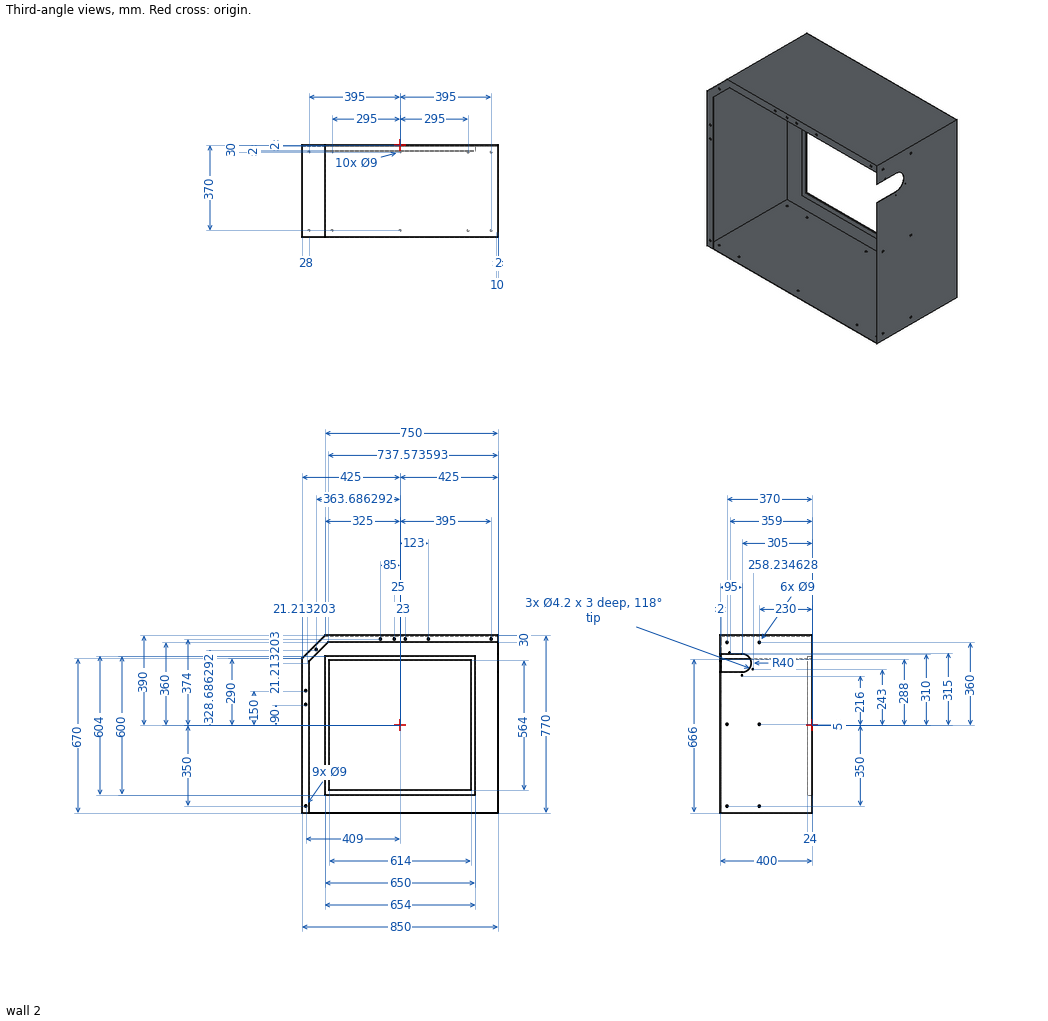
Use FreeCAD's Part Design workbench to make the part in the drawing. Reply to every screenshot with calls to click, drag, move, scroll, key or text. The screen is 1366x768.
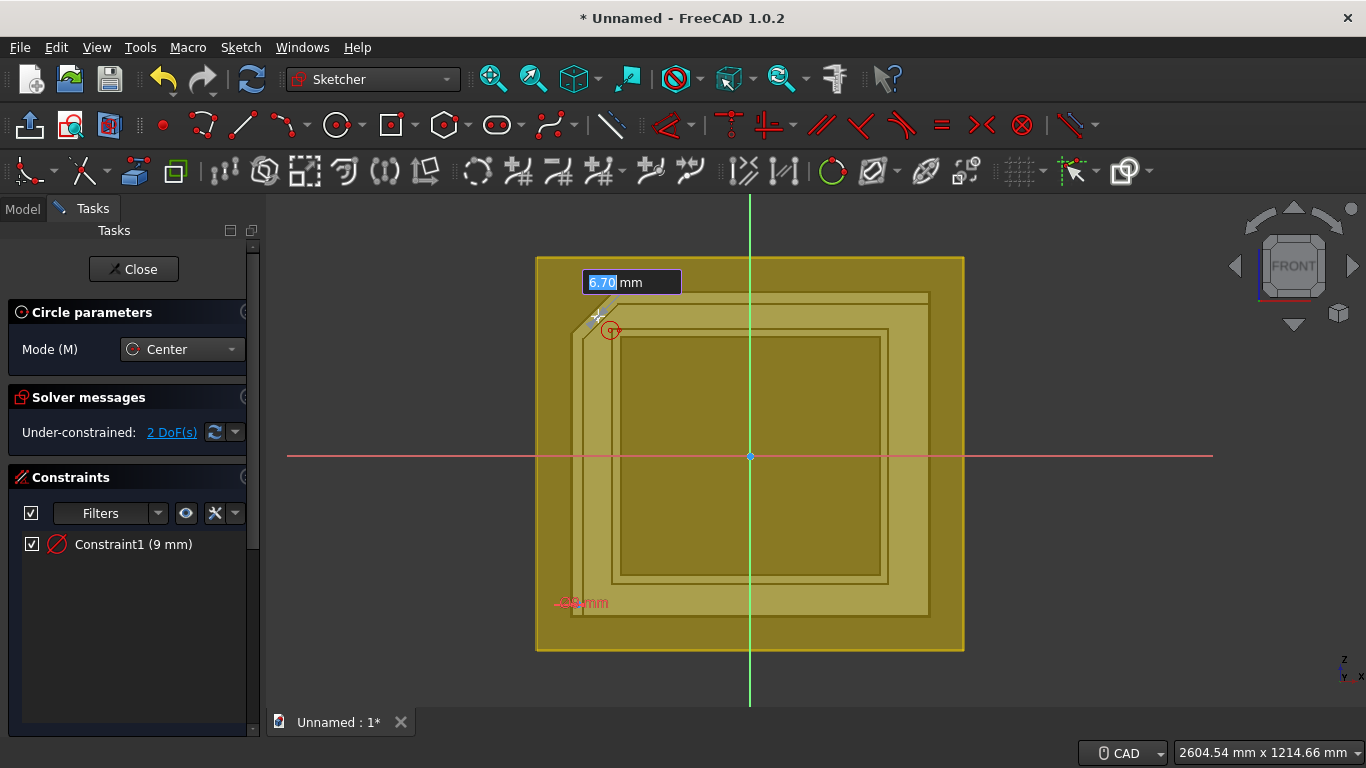
text(9)
key(Return)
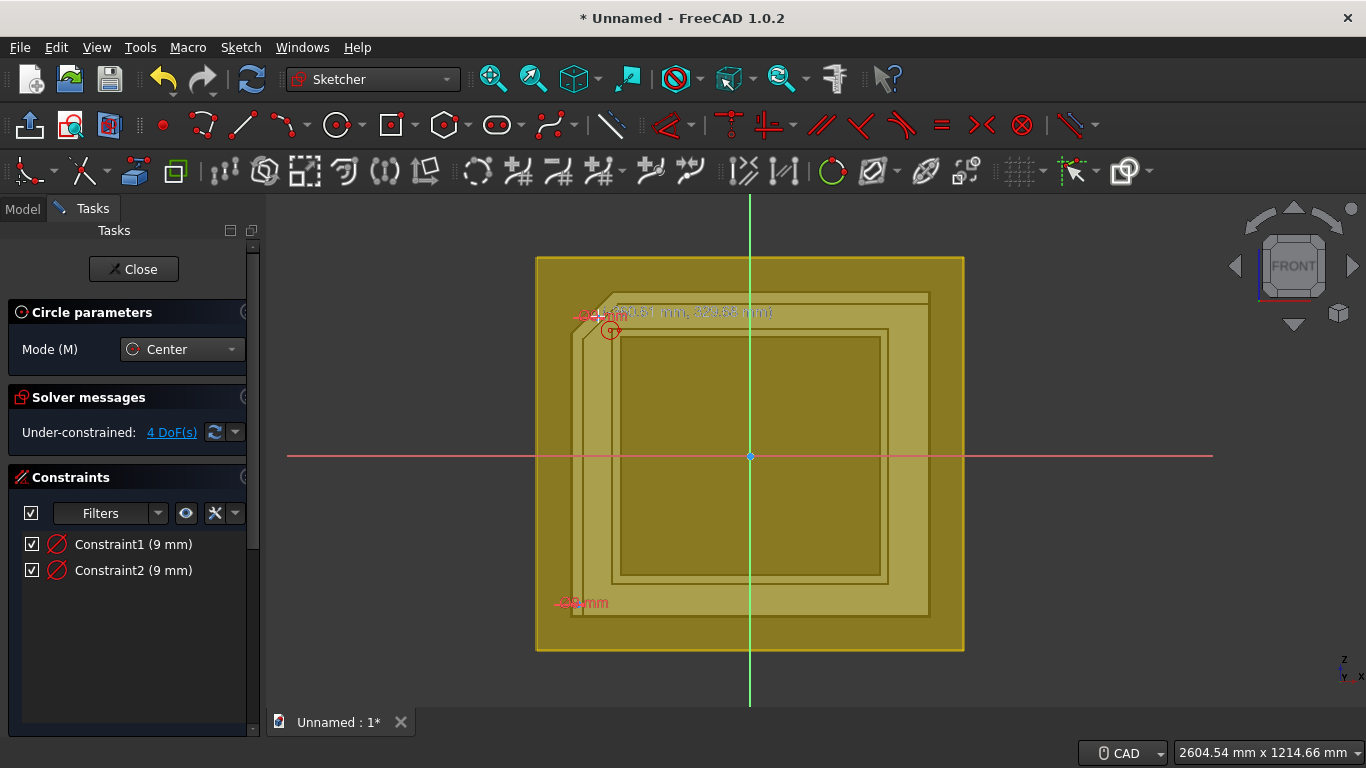
scroll(714, 298, up, 13)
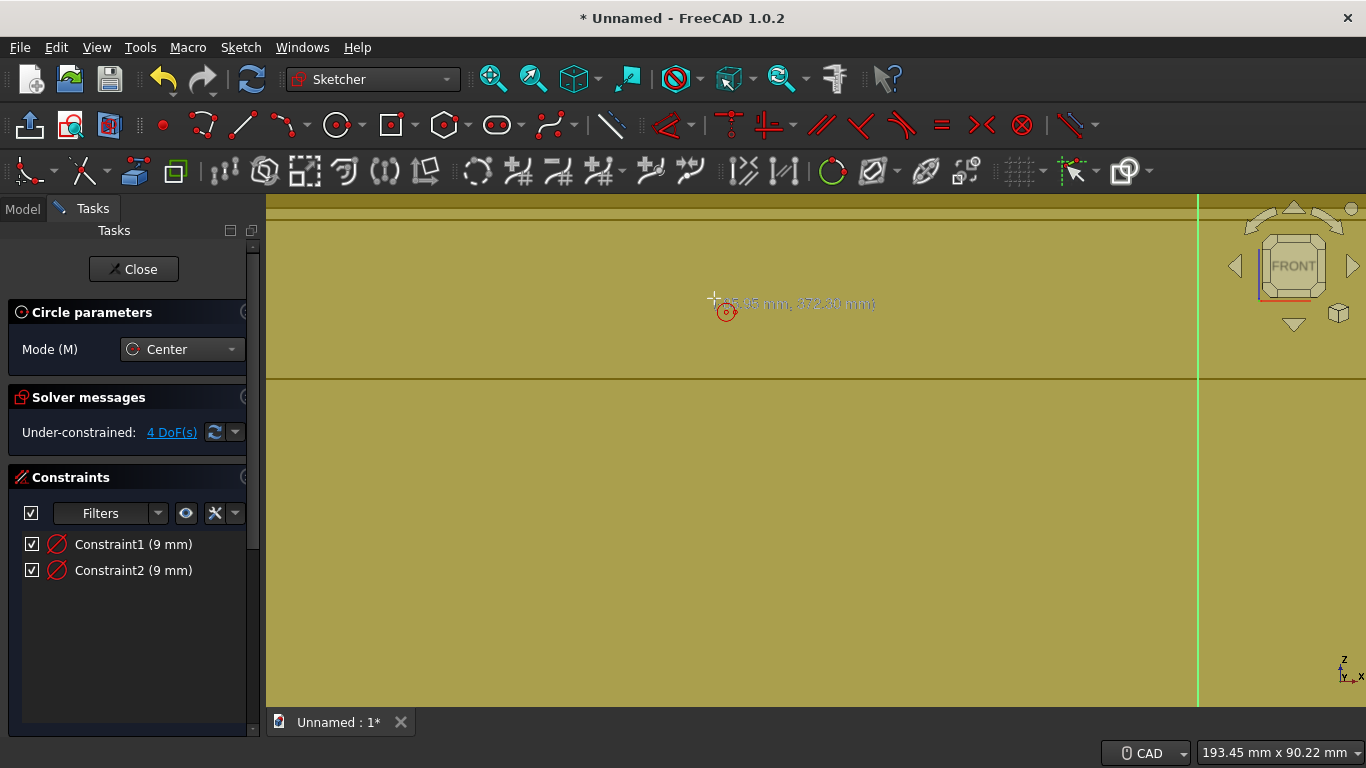
scroll(715, 297, down, 13)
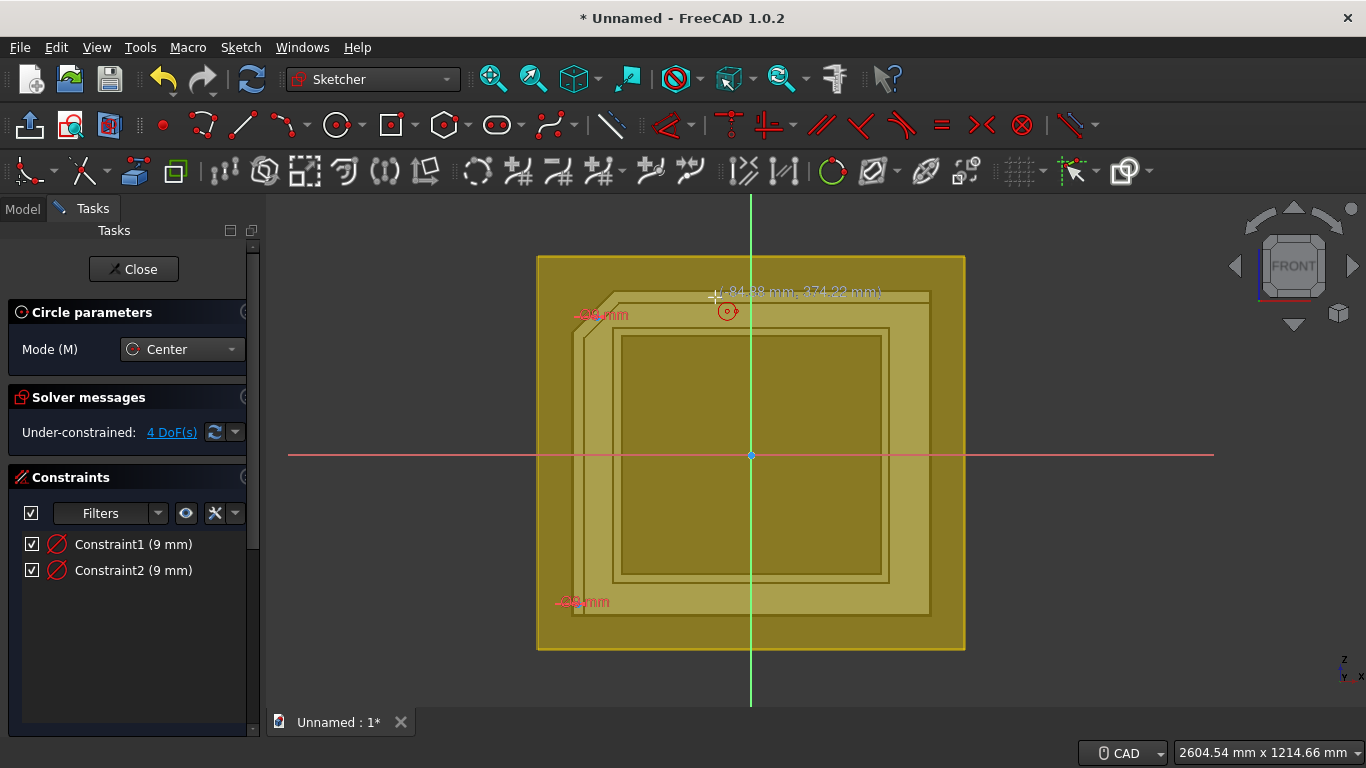
click(715, 297)
move(717, 296)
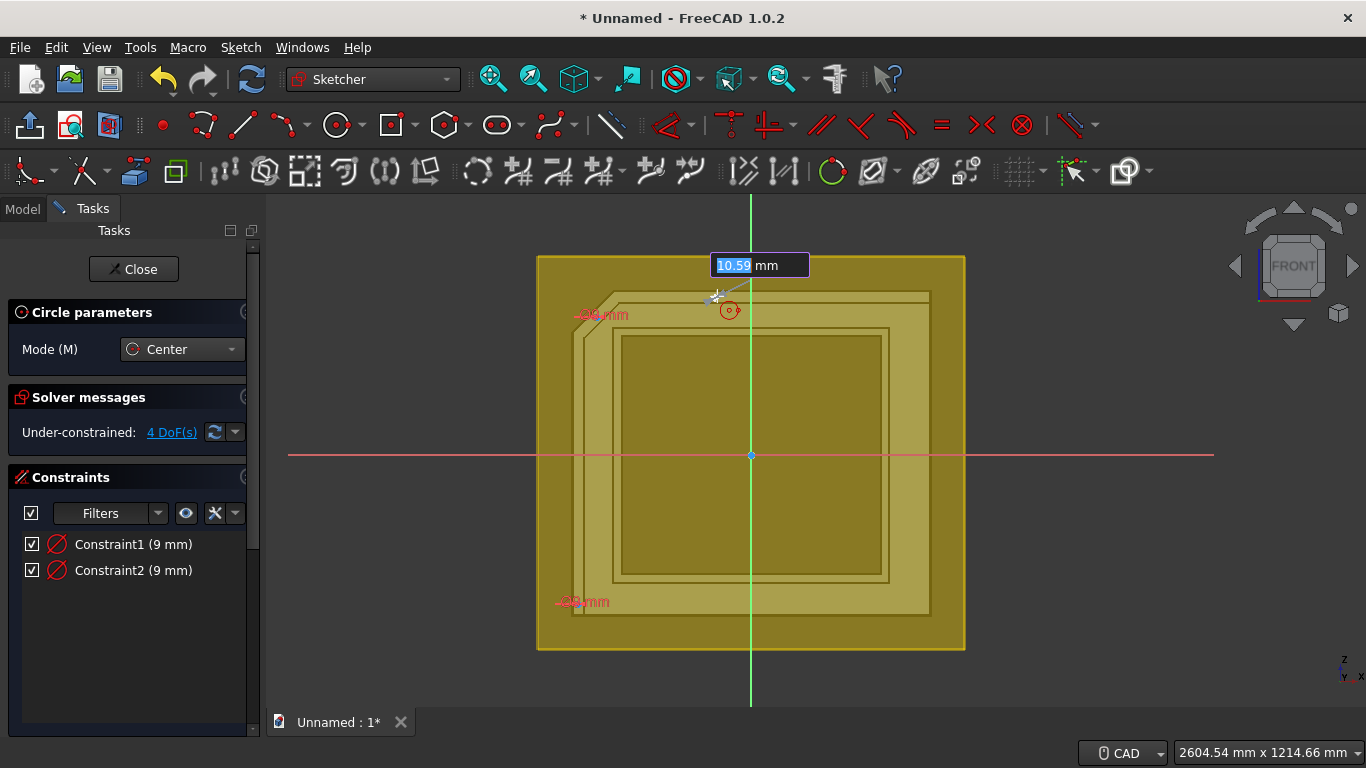
text(9)
key(Return)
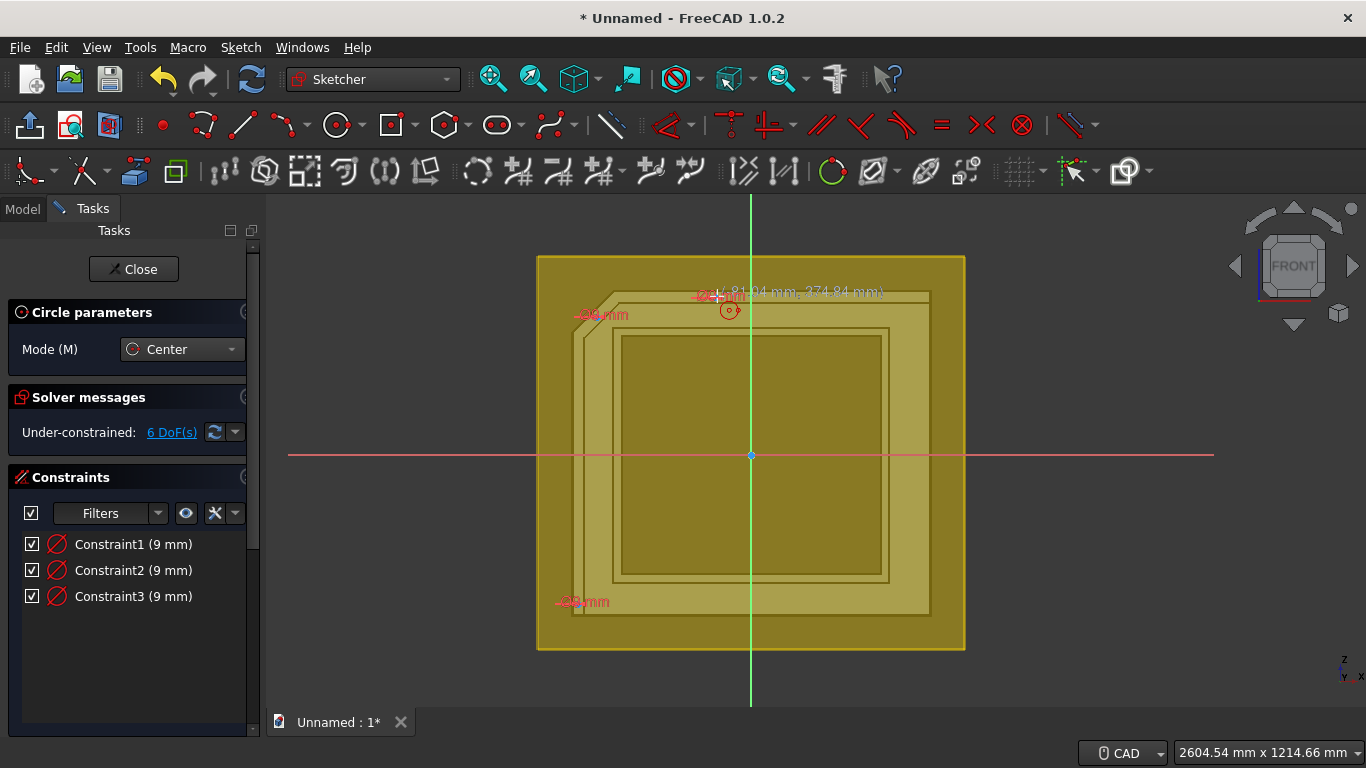
scroll(918, 297, up, 13)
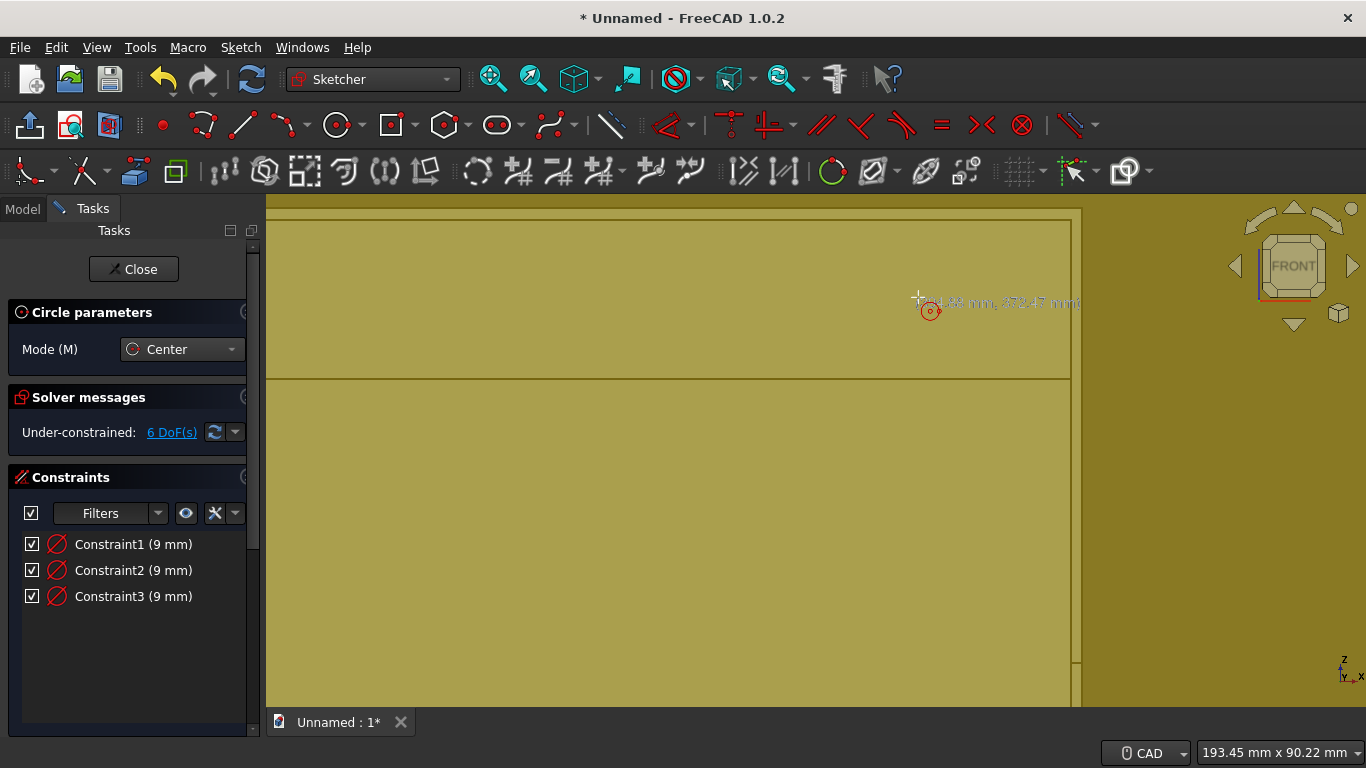
scroll(918, 297, down, 13)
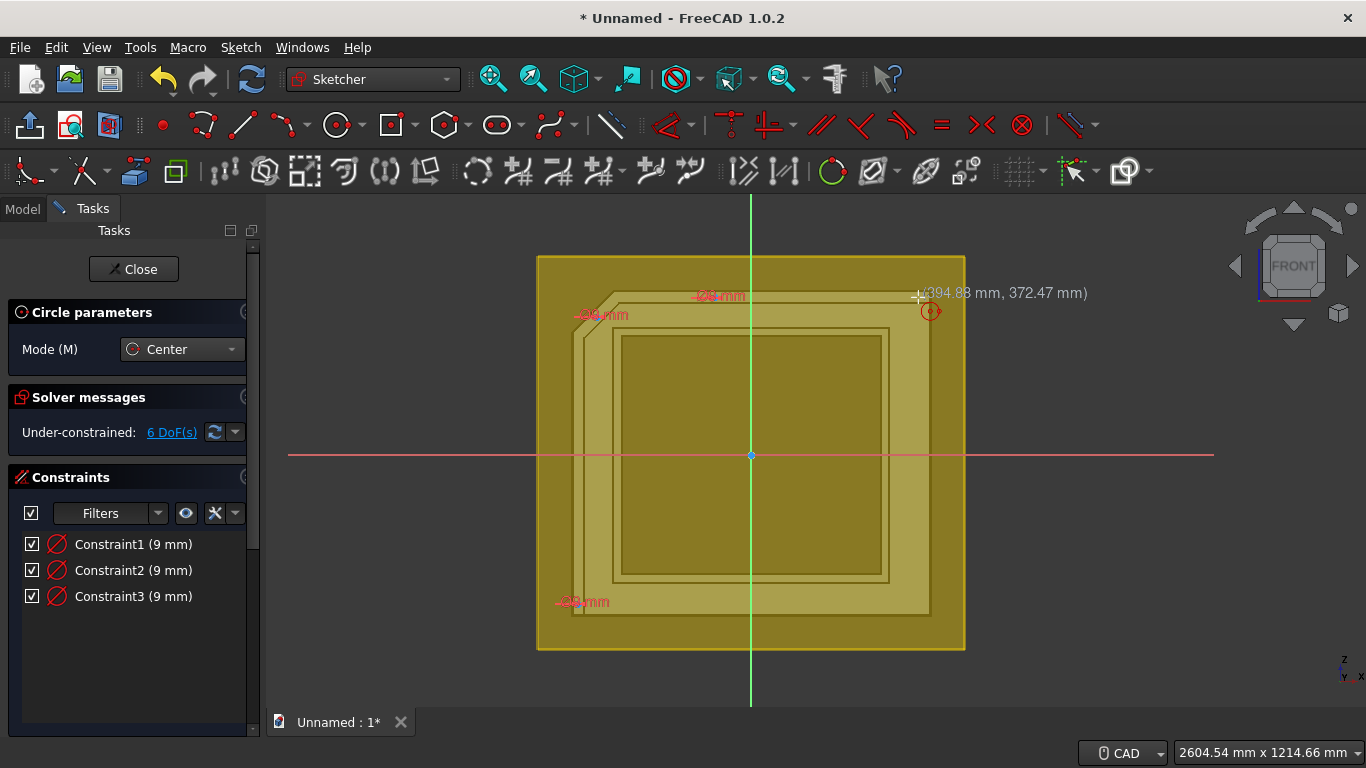
click(918, 297)
move(919, 296)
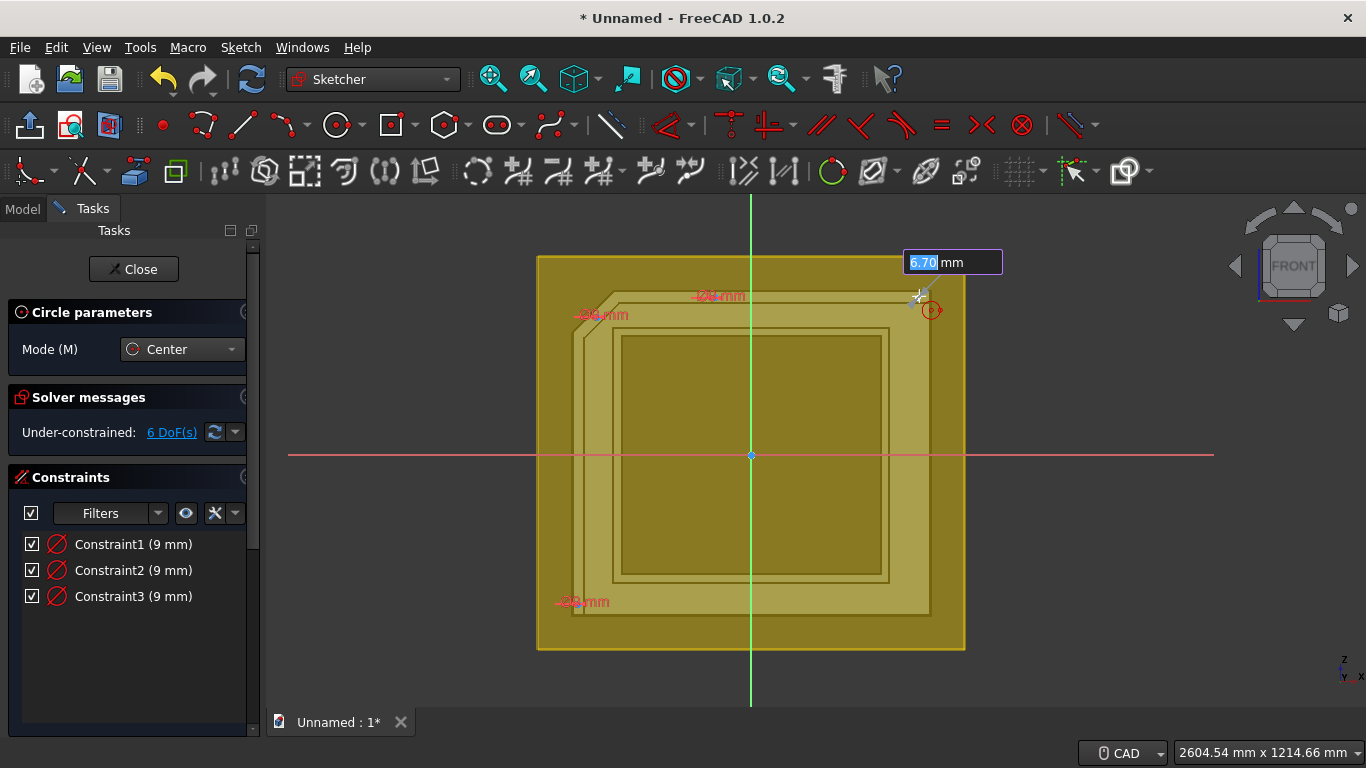
text(9)
key(Return)